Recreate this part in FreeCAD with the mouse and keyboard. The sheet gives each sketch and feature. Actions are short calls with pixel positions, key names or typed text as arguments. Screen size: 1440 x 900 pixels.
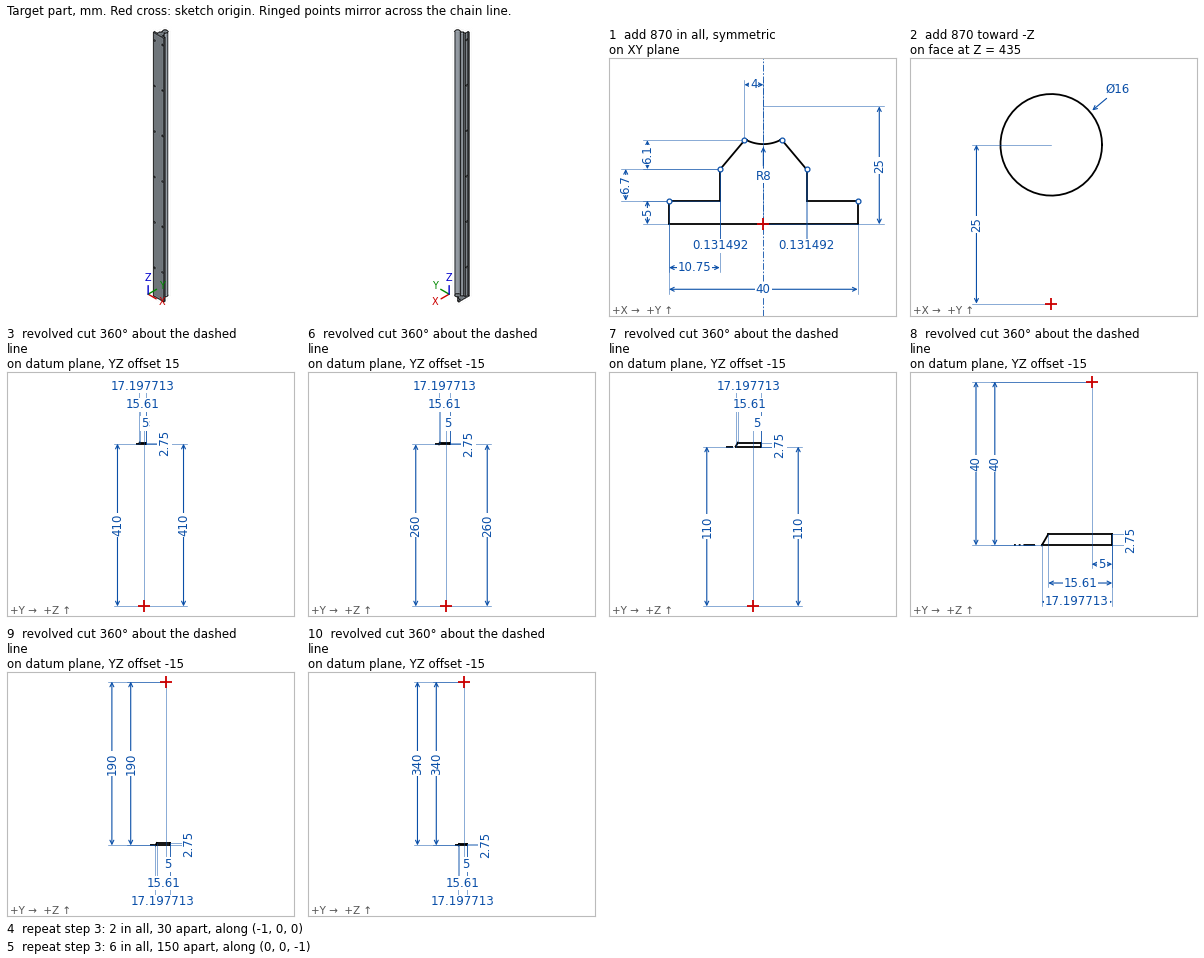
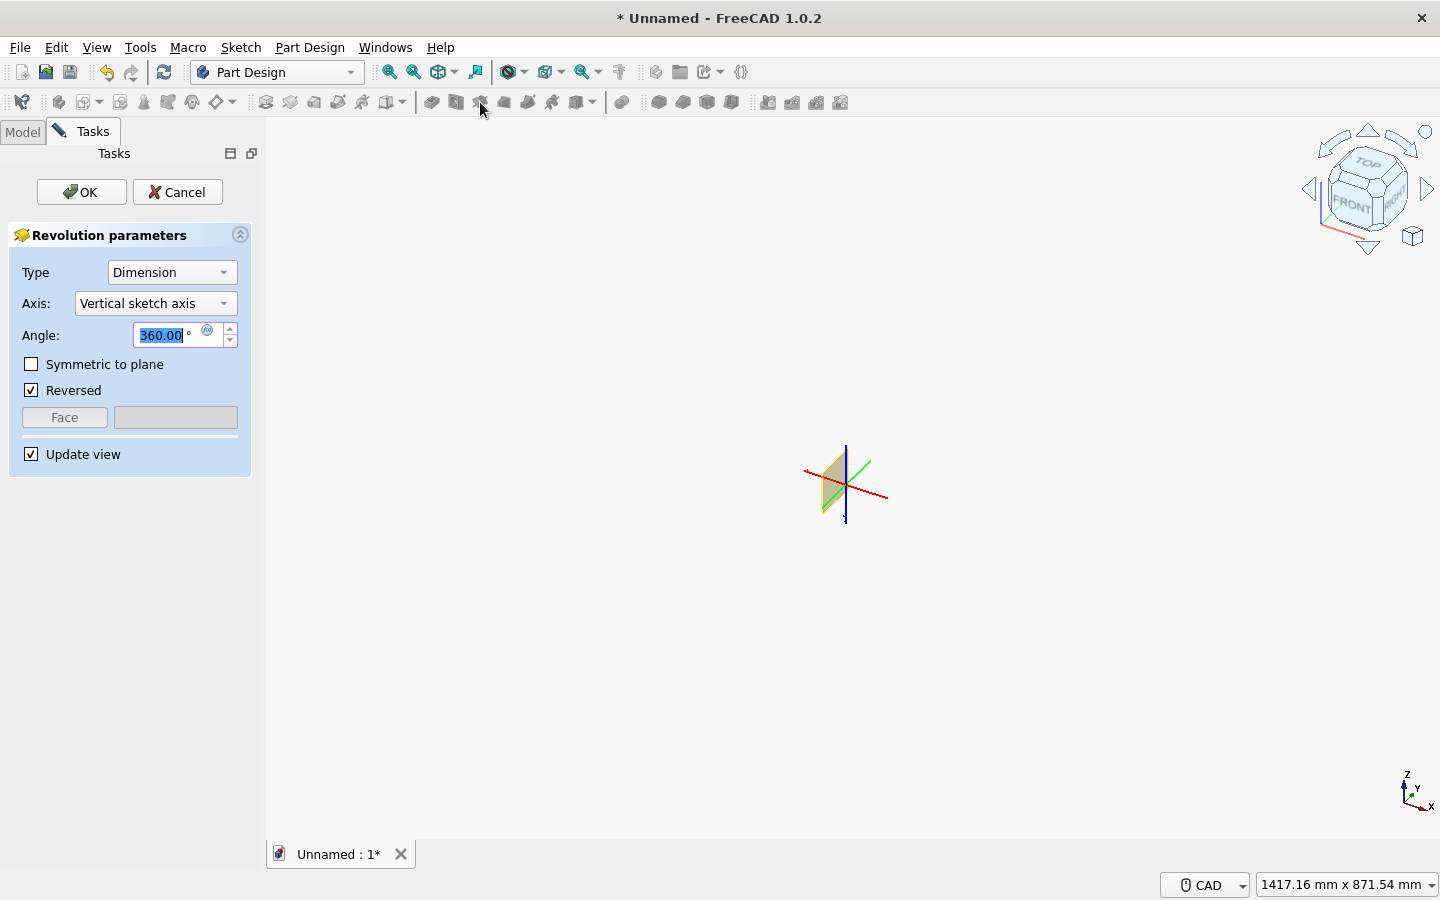
click(156, 304)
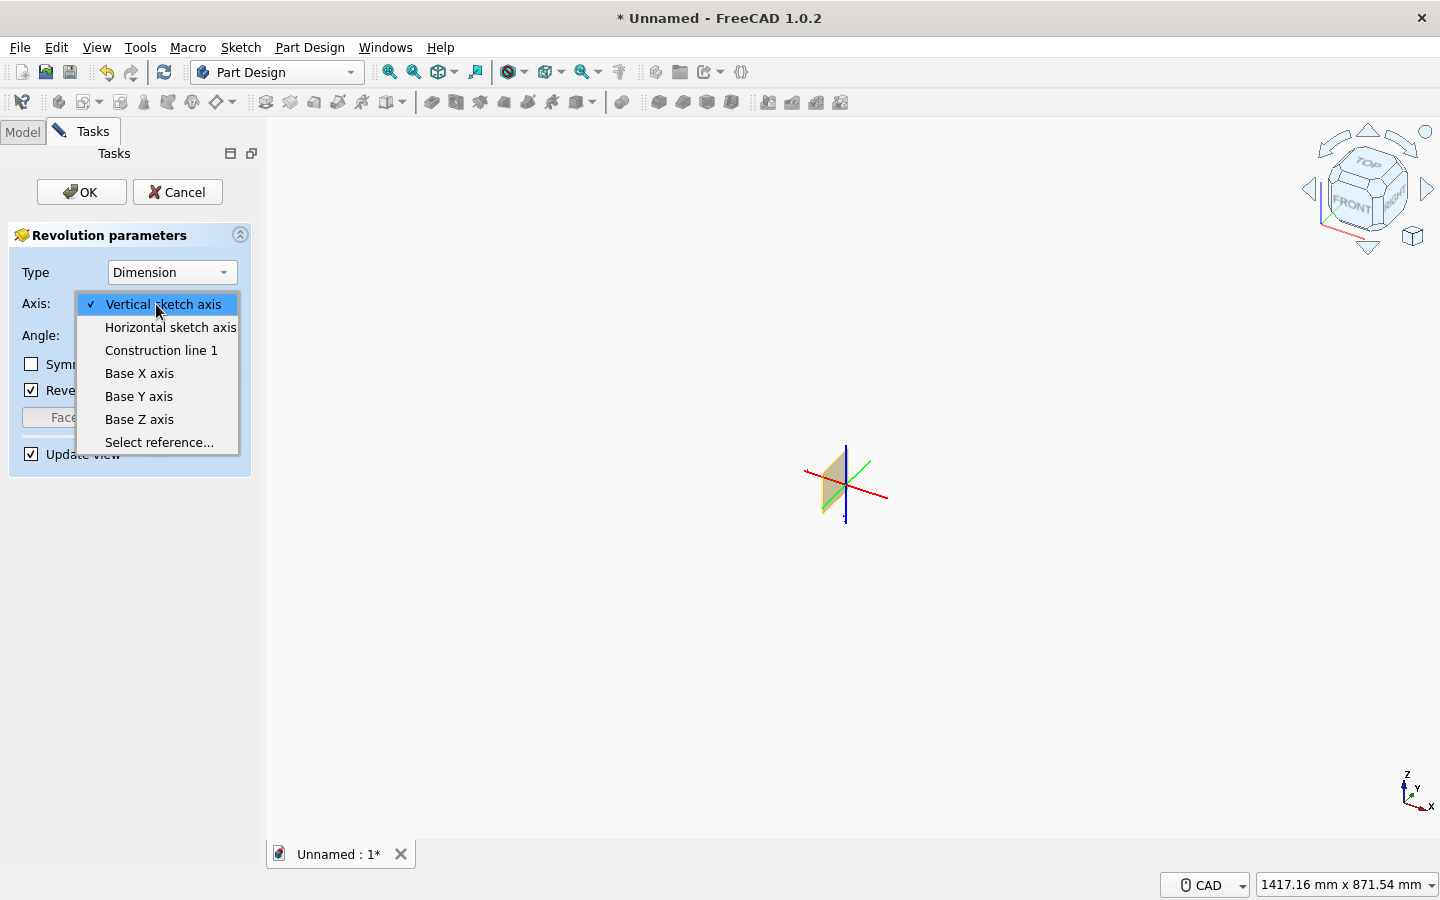
click(156, 350)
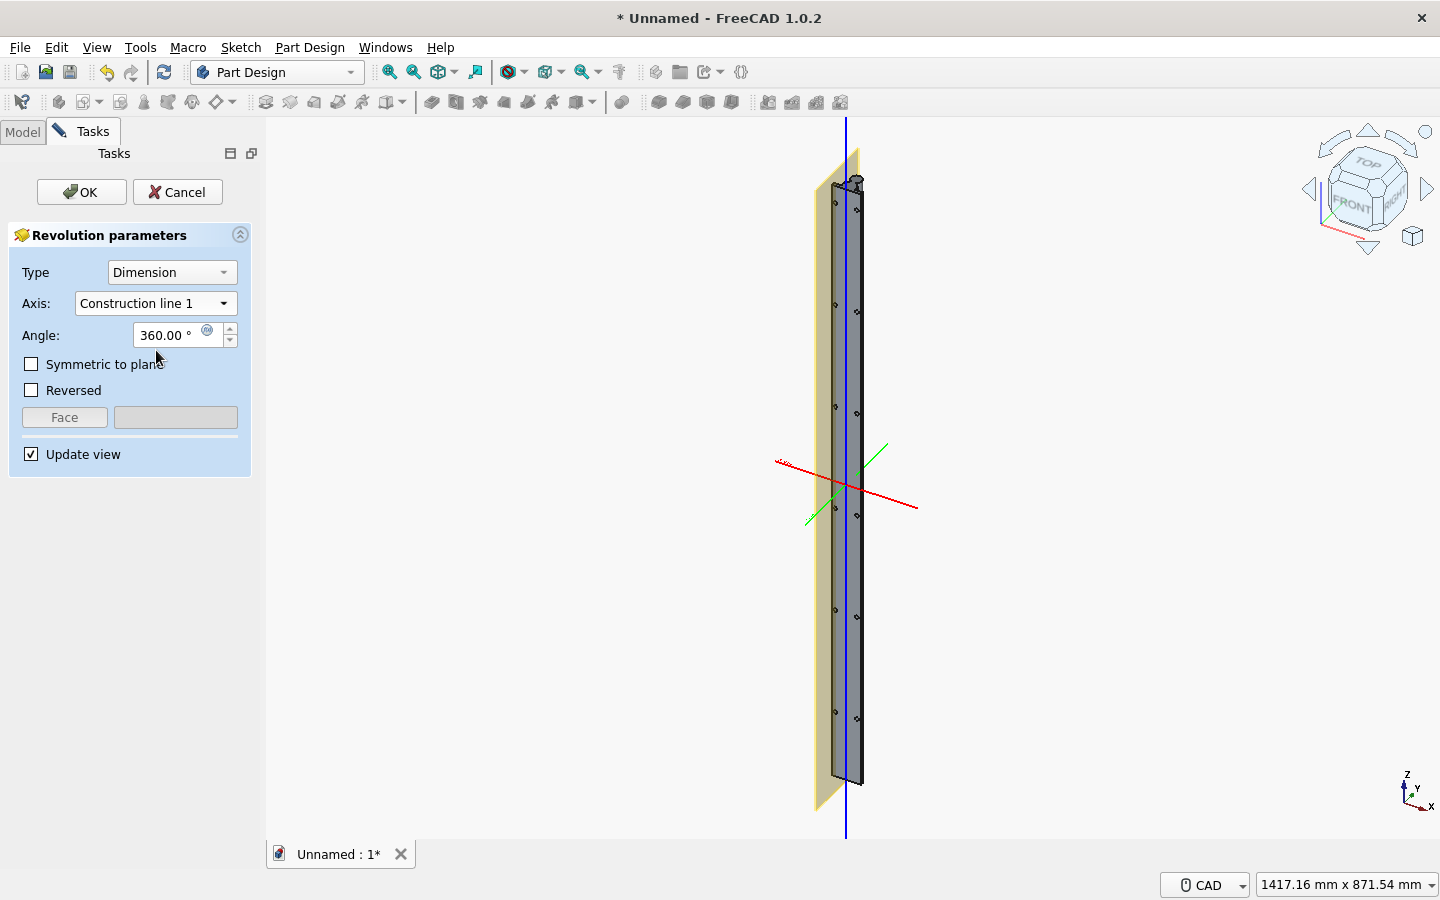
click(82, 192)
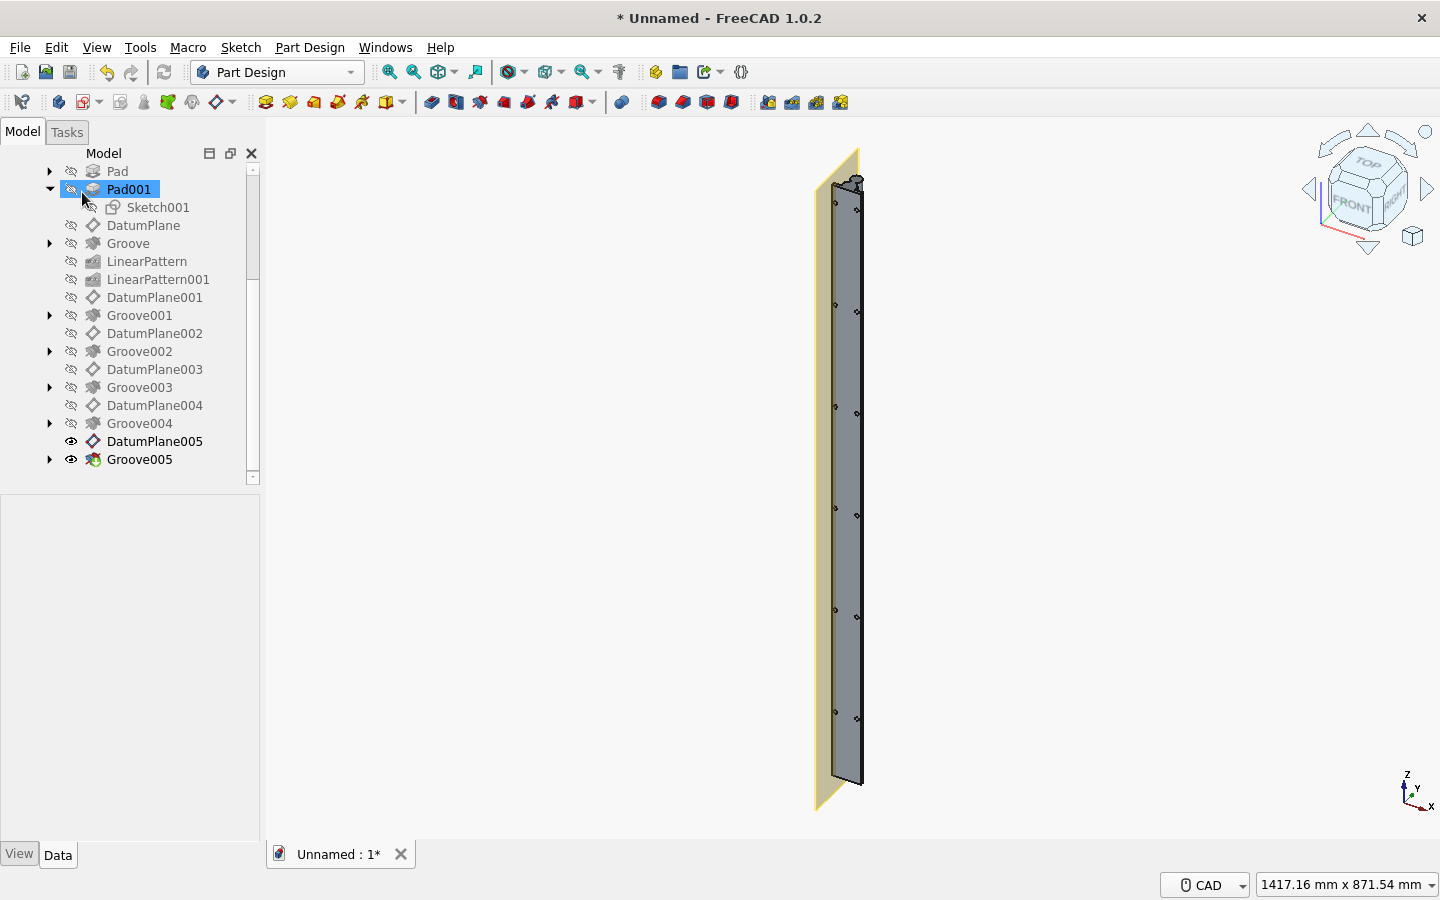
click(116, 441)
key(space)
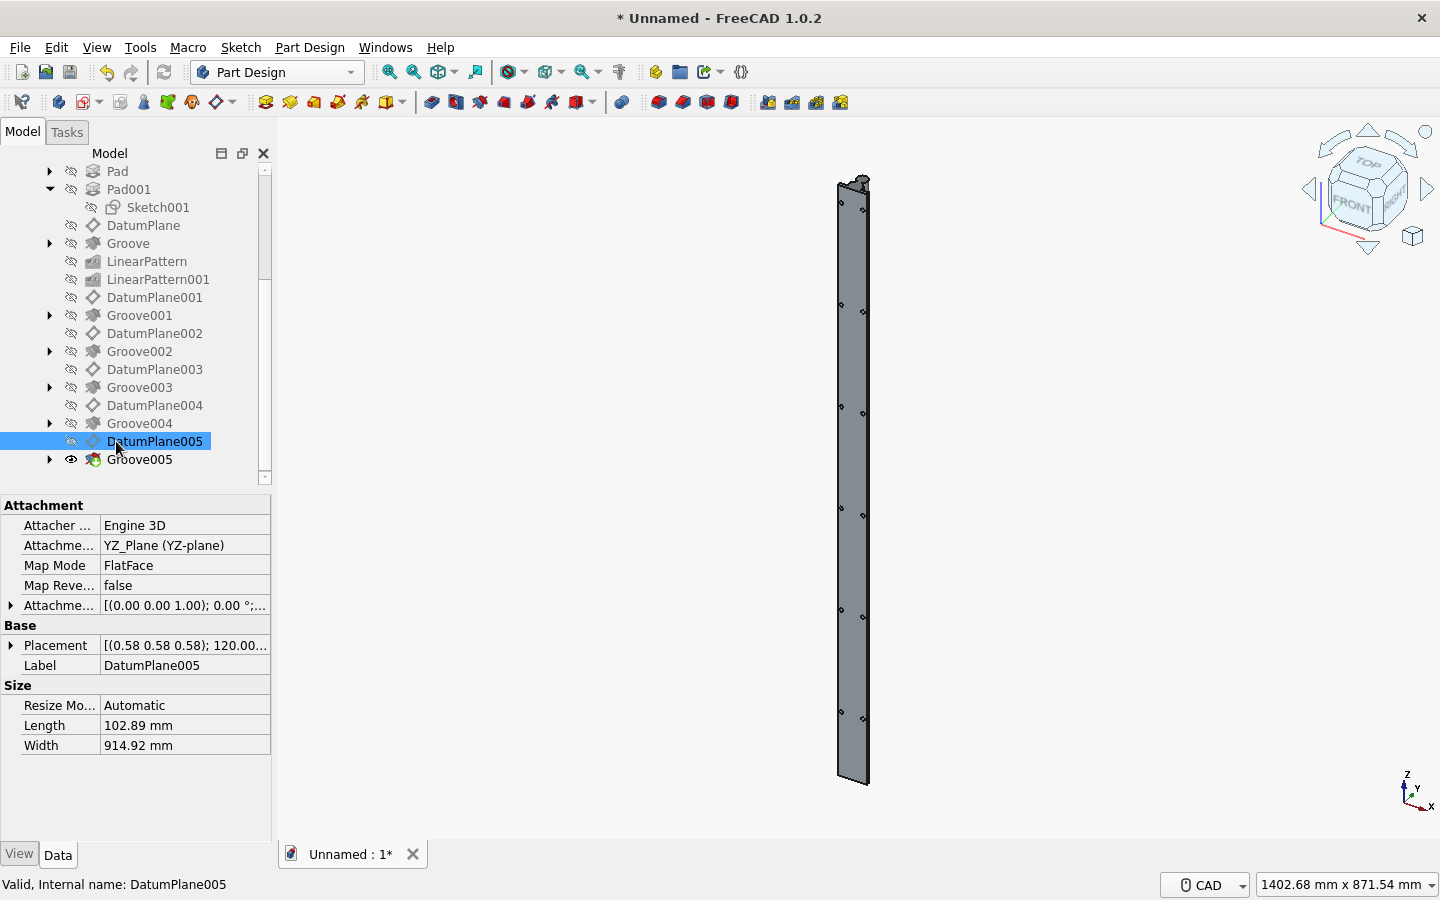
key(0)